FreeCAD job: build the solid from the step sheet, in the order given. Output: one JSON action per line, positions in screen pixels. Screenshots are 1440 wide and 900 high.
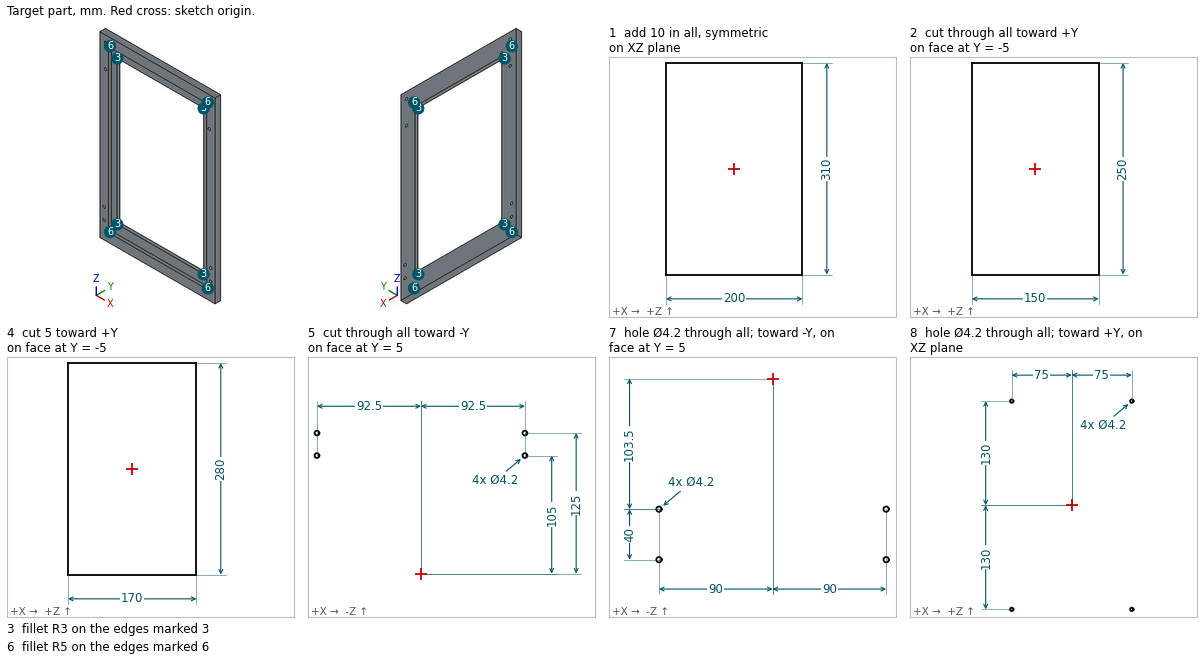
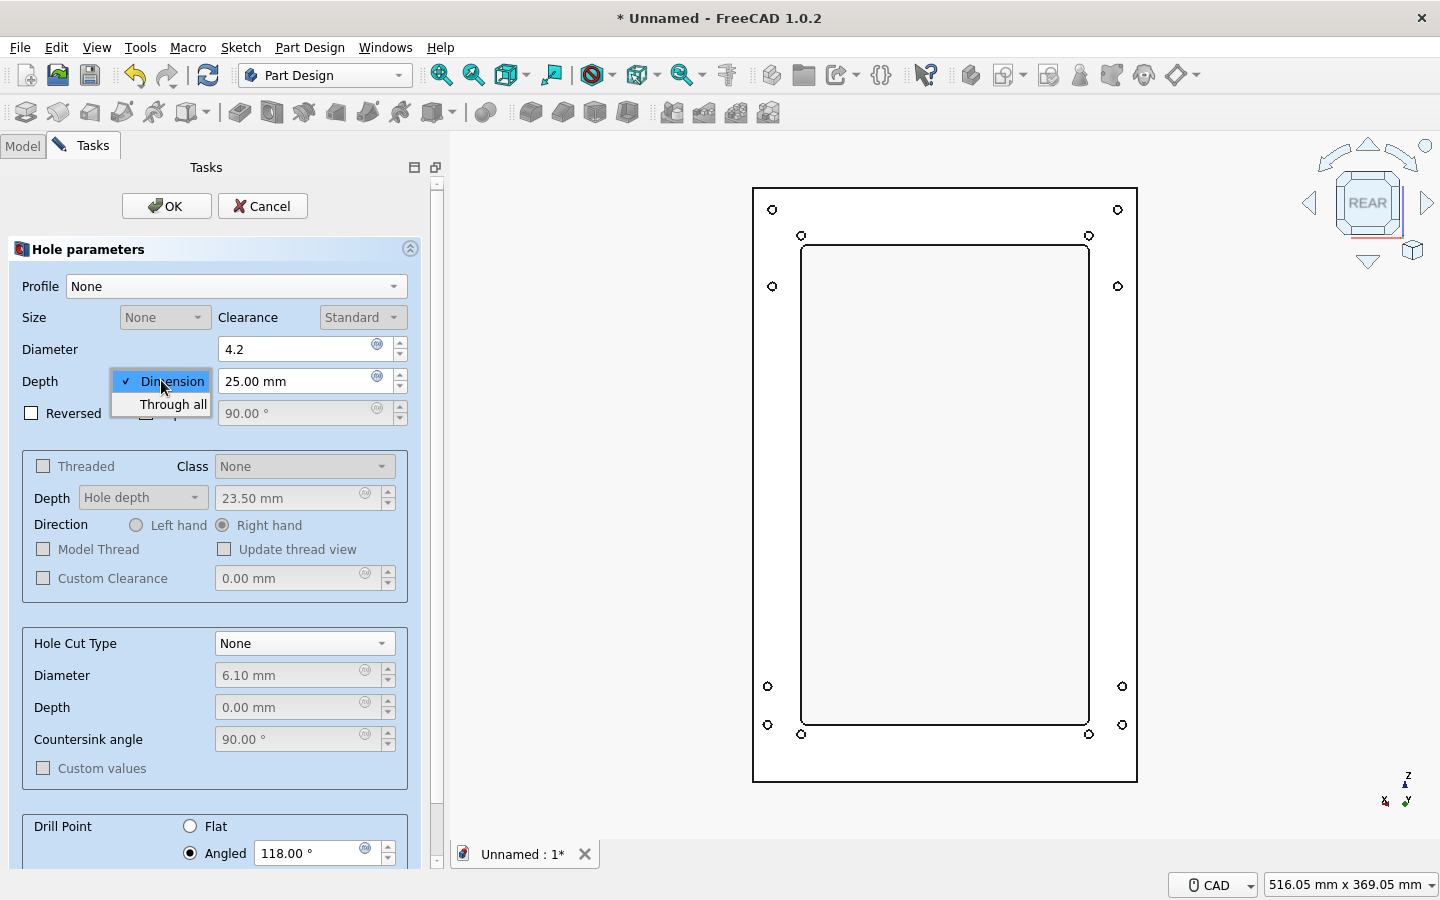
{"action": "left_click", "coordinate": [160, 404]}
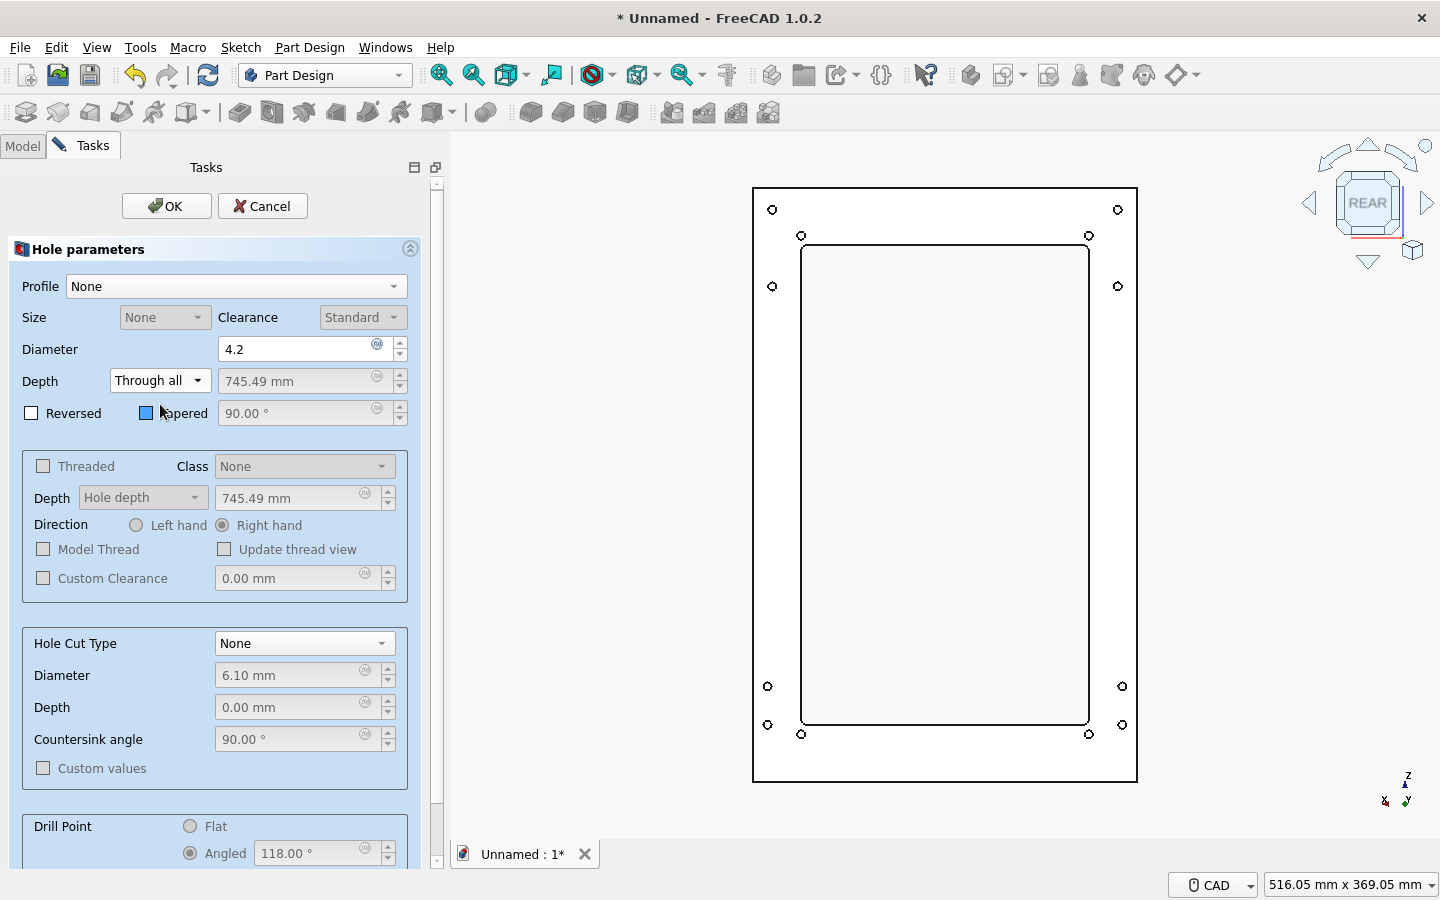
{"action": "left_click", "coordinate": [167, 206]}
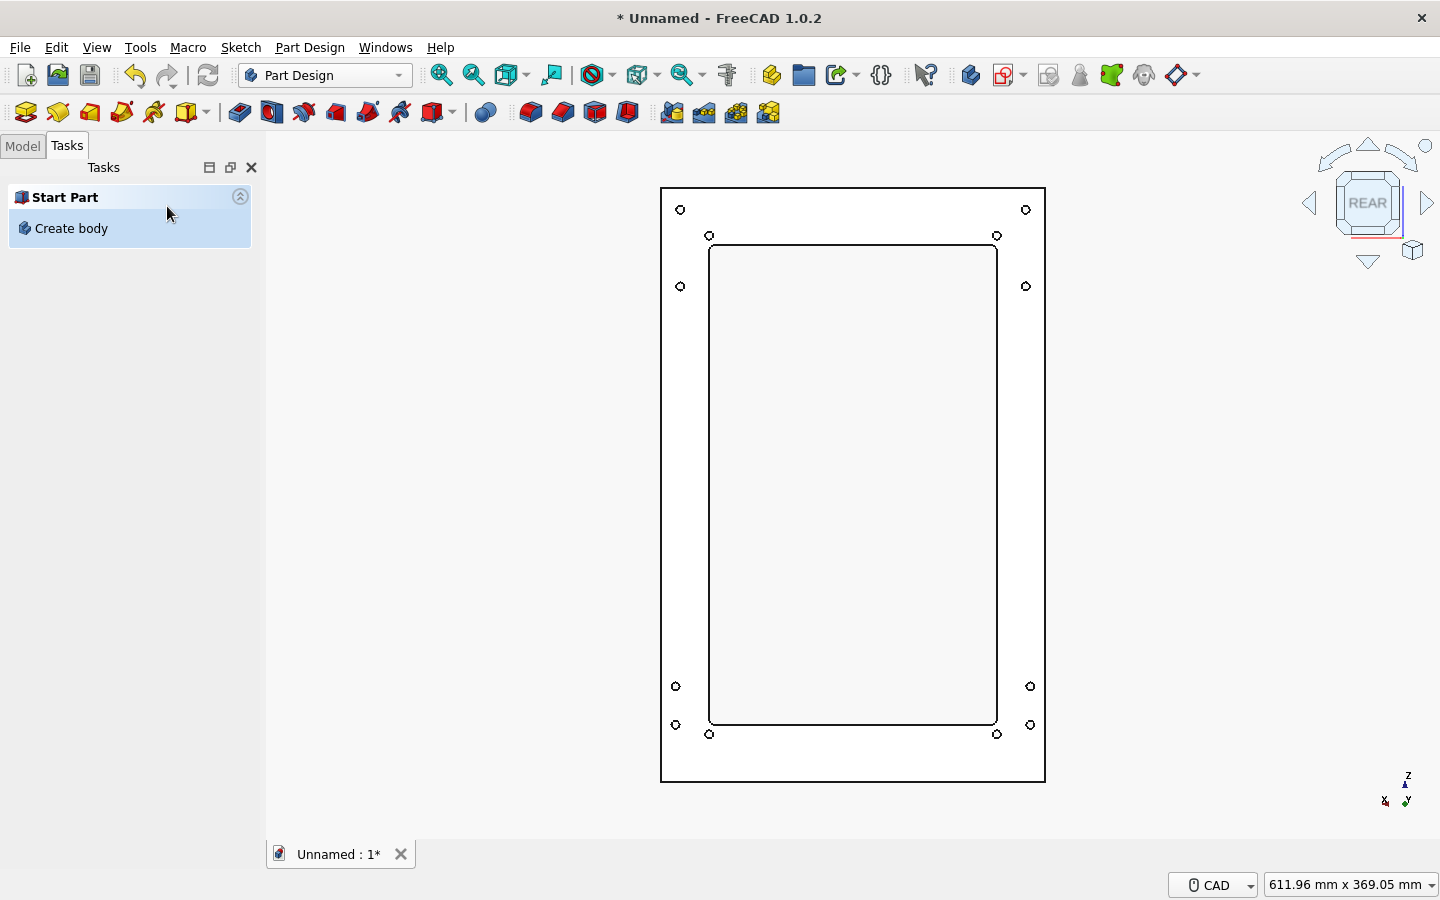
{"action": "key", "text": "0"}